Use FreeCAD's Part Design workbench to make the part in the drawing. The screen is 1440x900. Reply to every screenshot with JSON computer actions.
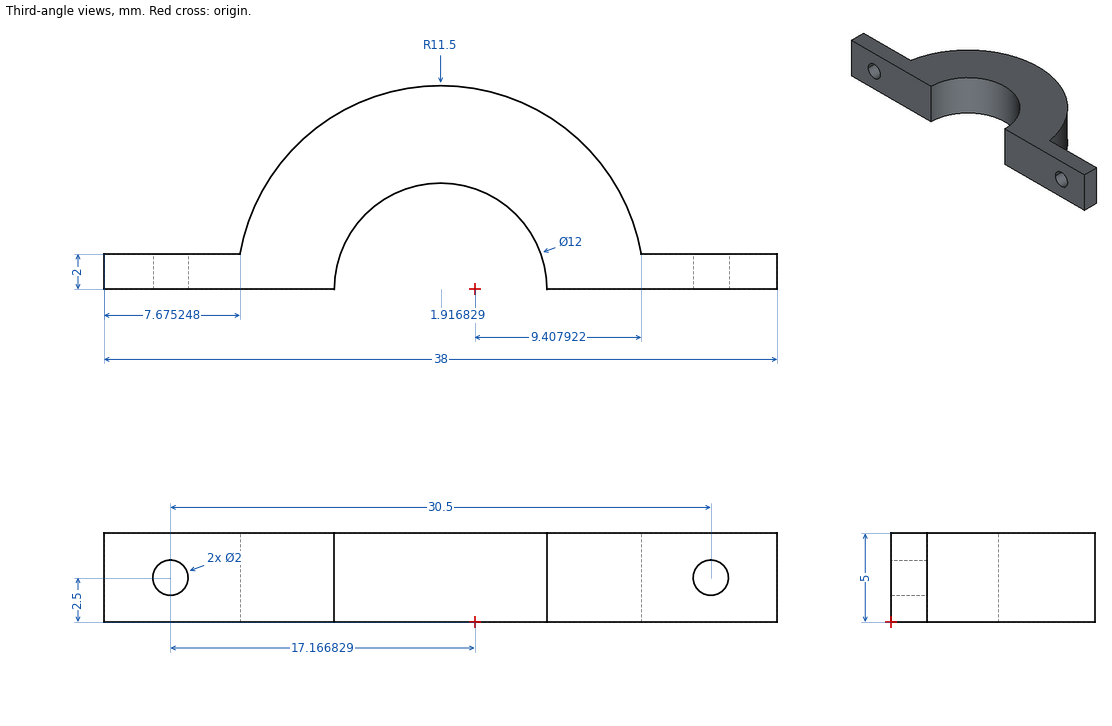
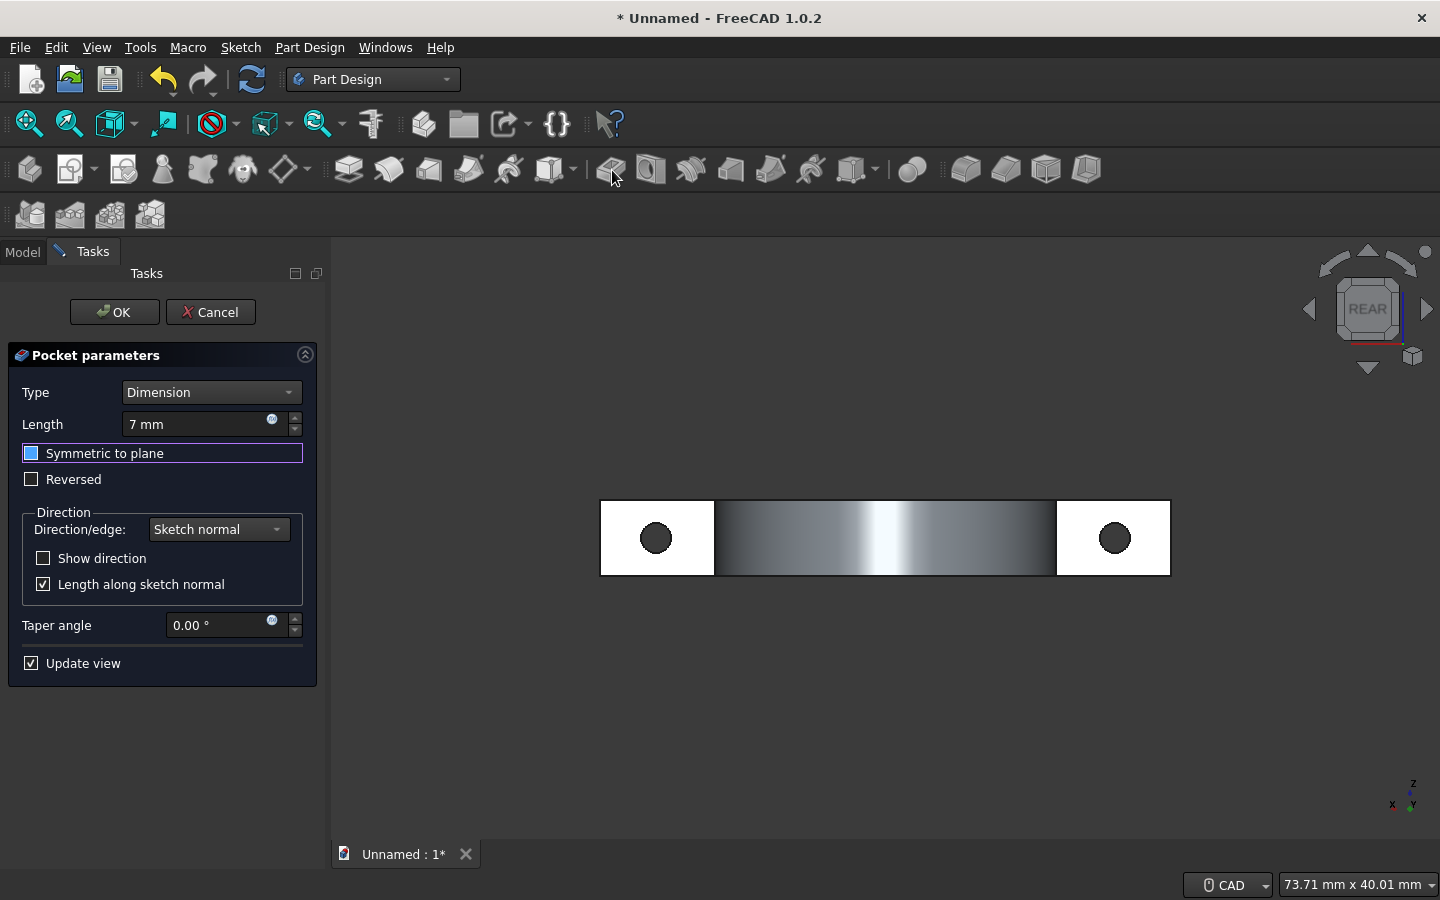
{"action": "left_click", "coordinate": [115, 312]}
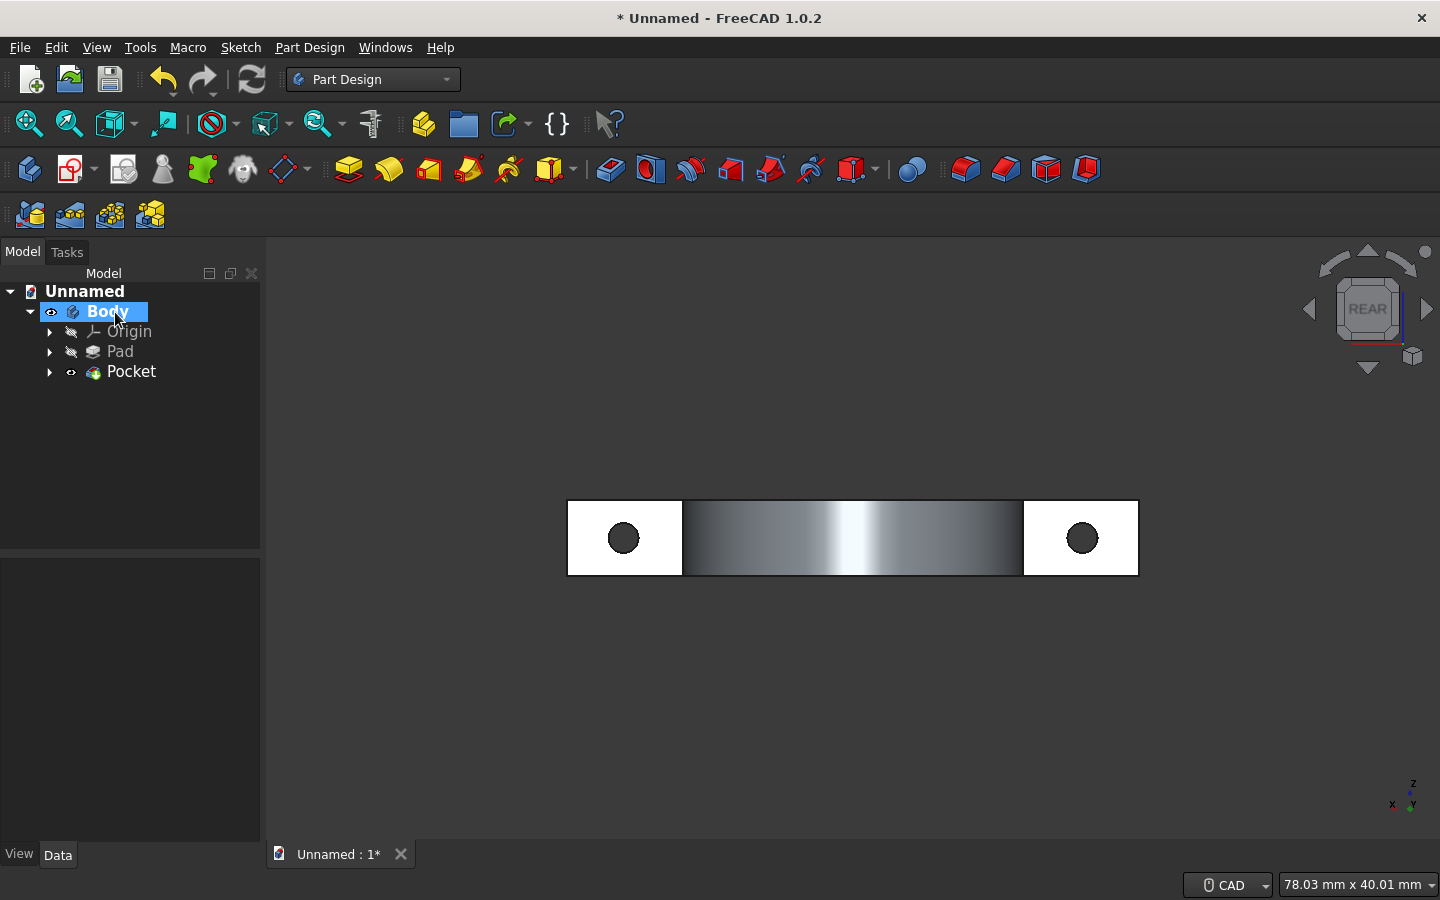
{"action": "key", "text": "0"}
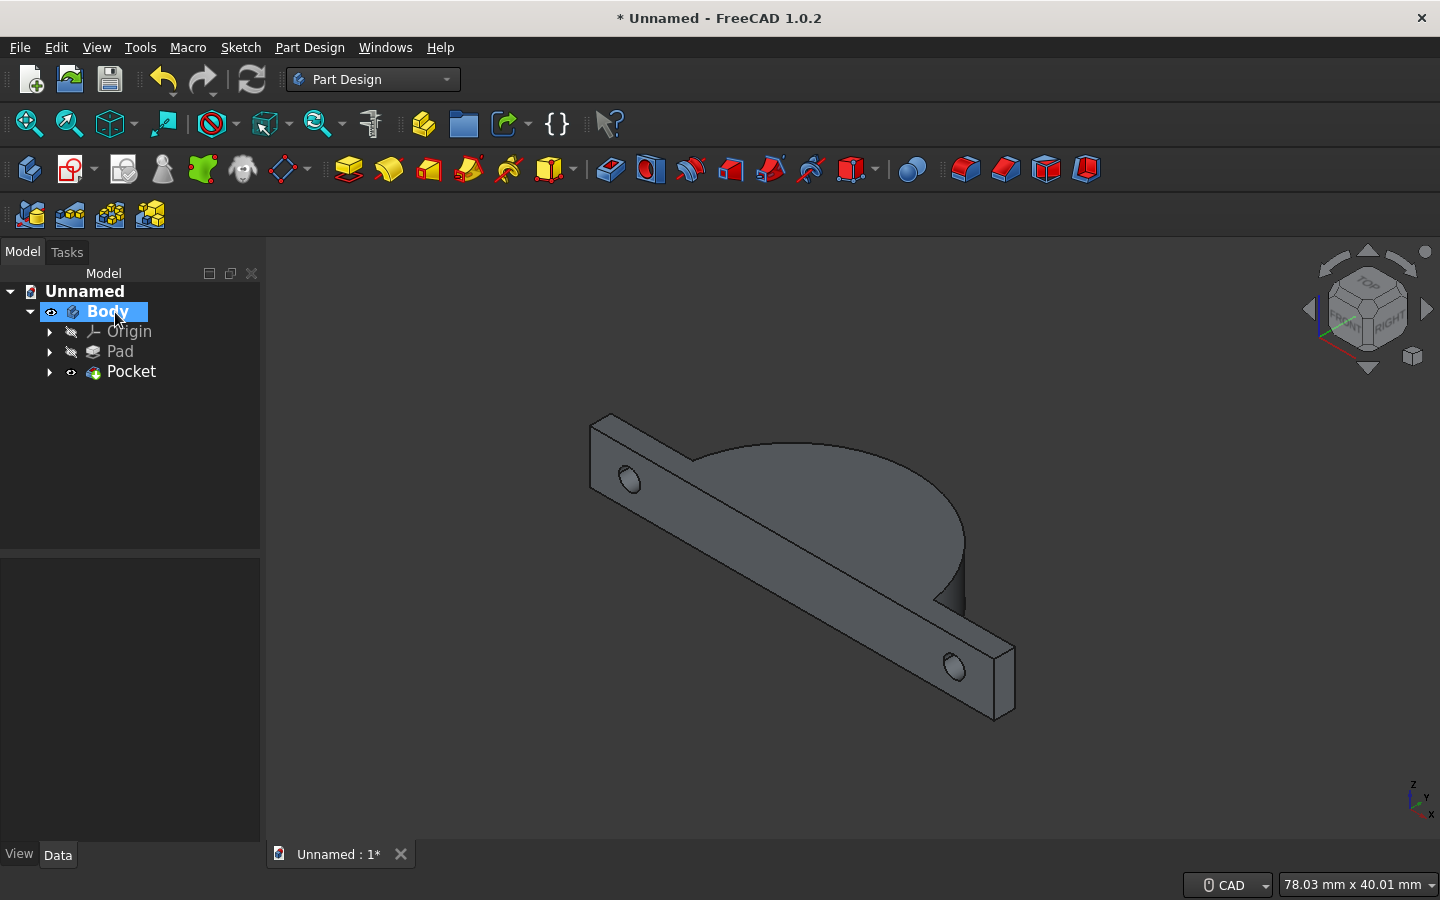
{"action": "left_click", "coordinate": [853, 506]}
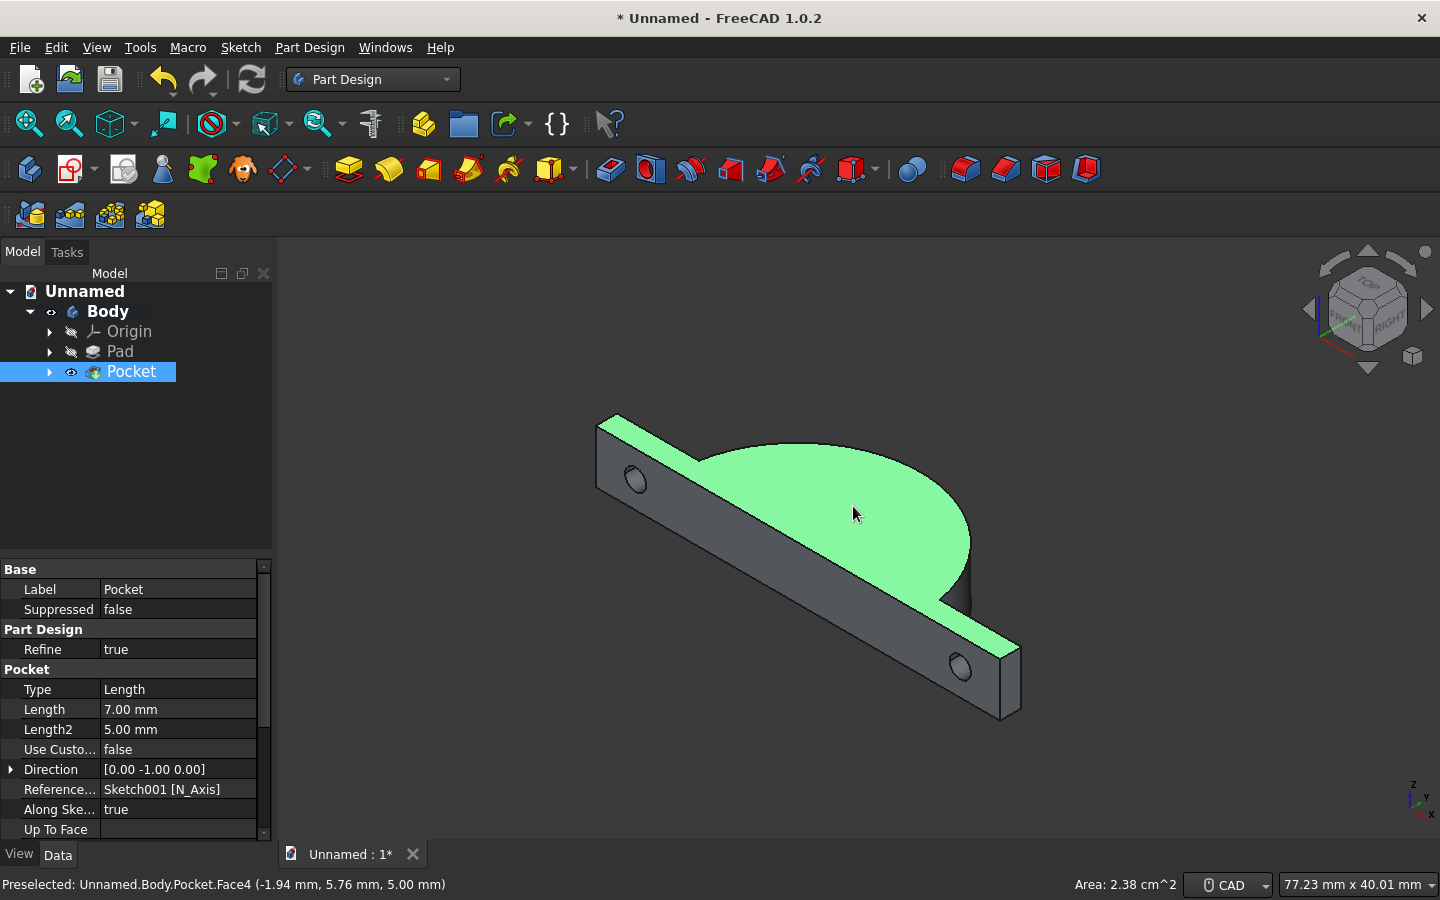
{"action": "left_click", "coordinate": [70, 170]}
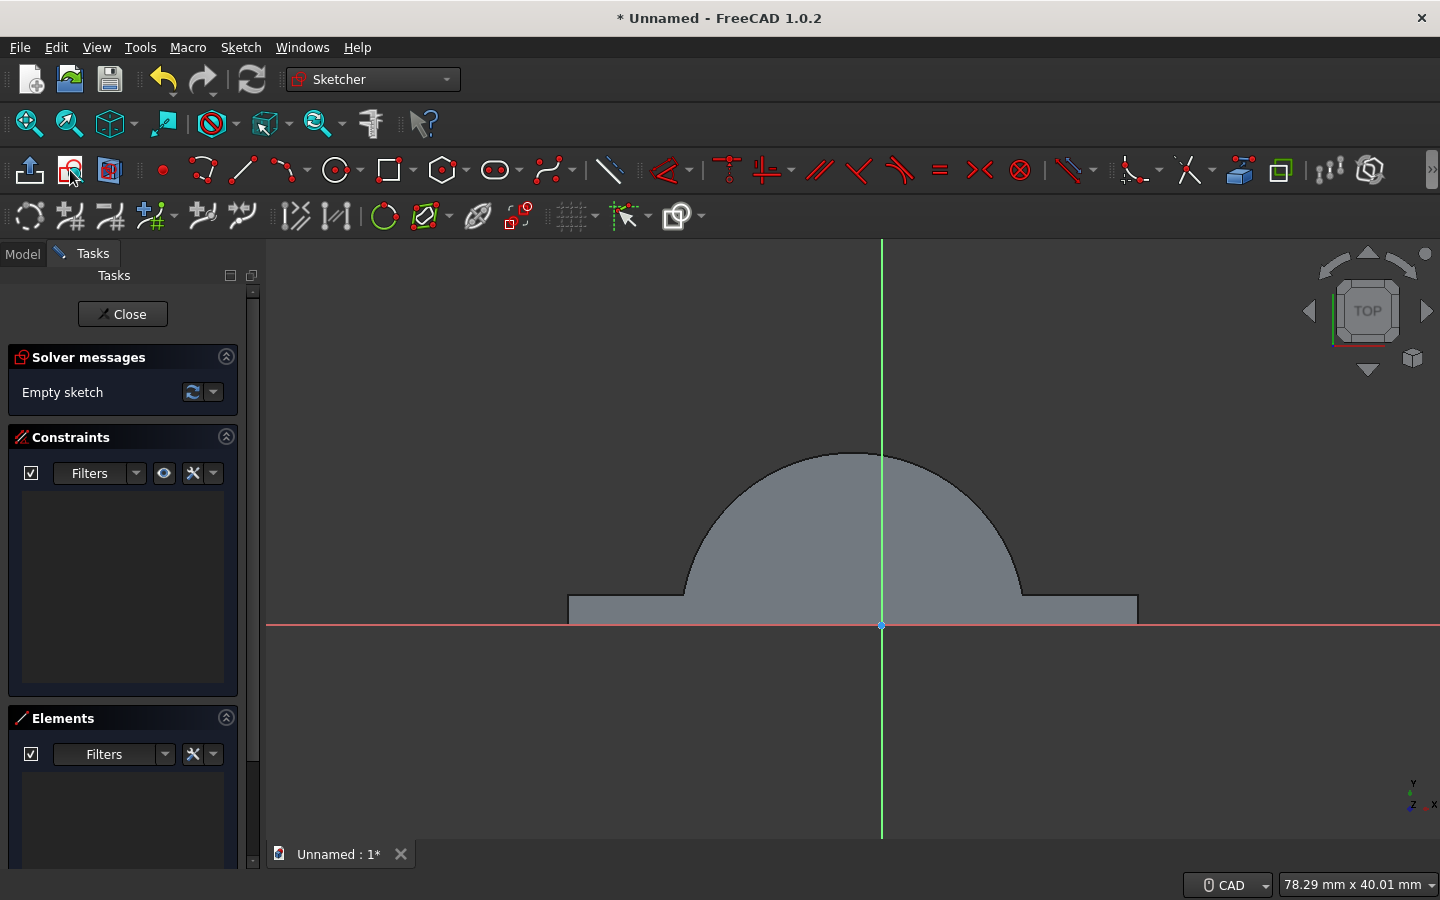
{"action": "scroll", "coordinate": [909, 695], "scroll_direction": "up", "scroll_amount": 4}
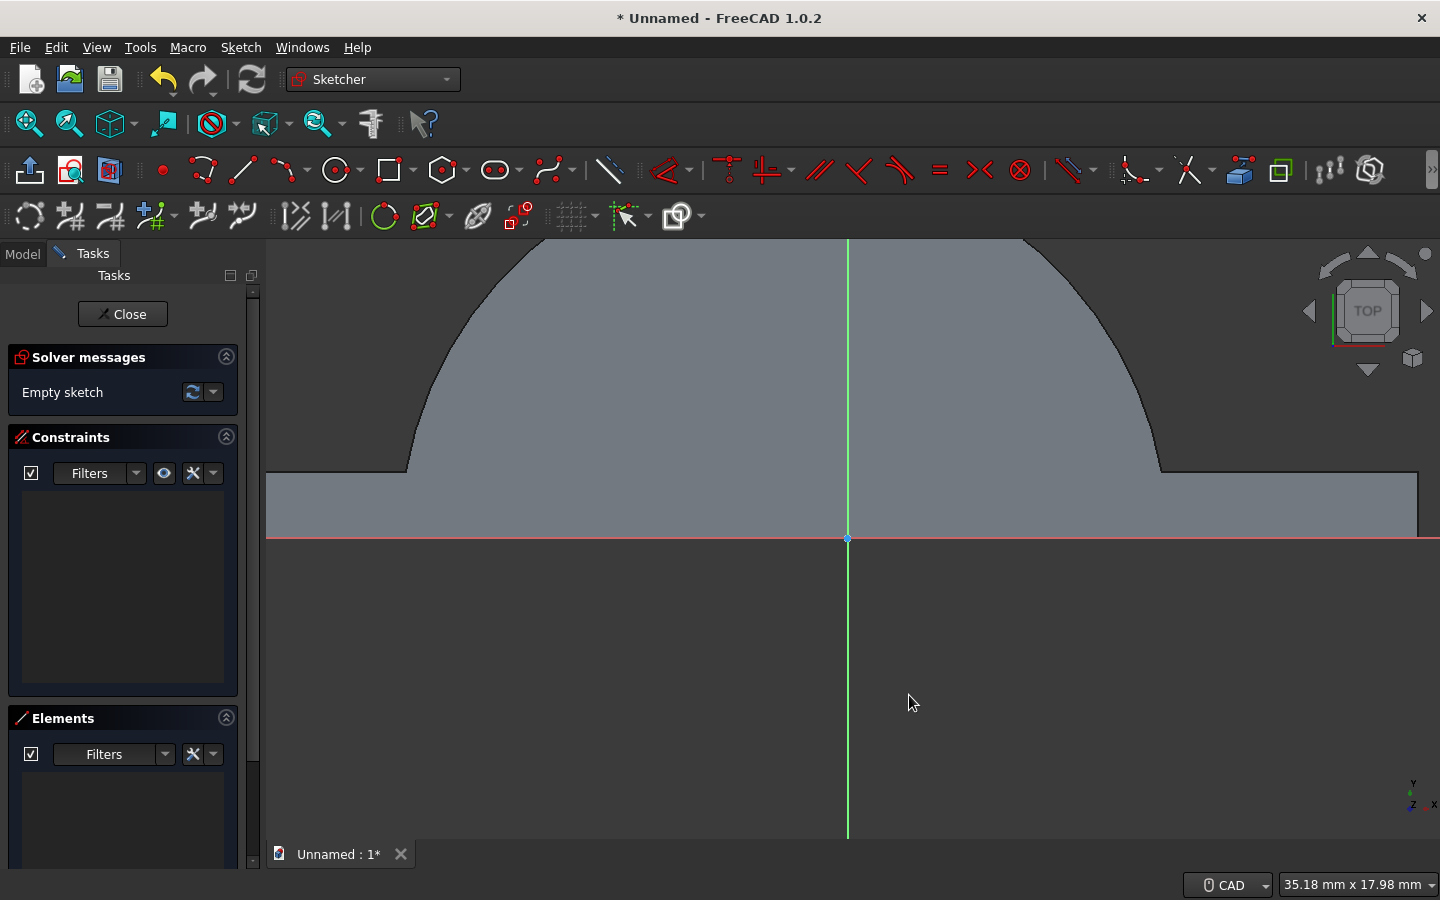
{"action": "key", "text": "g c"}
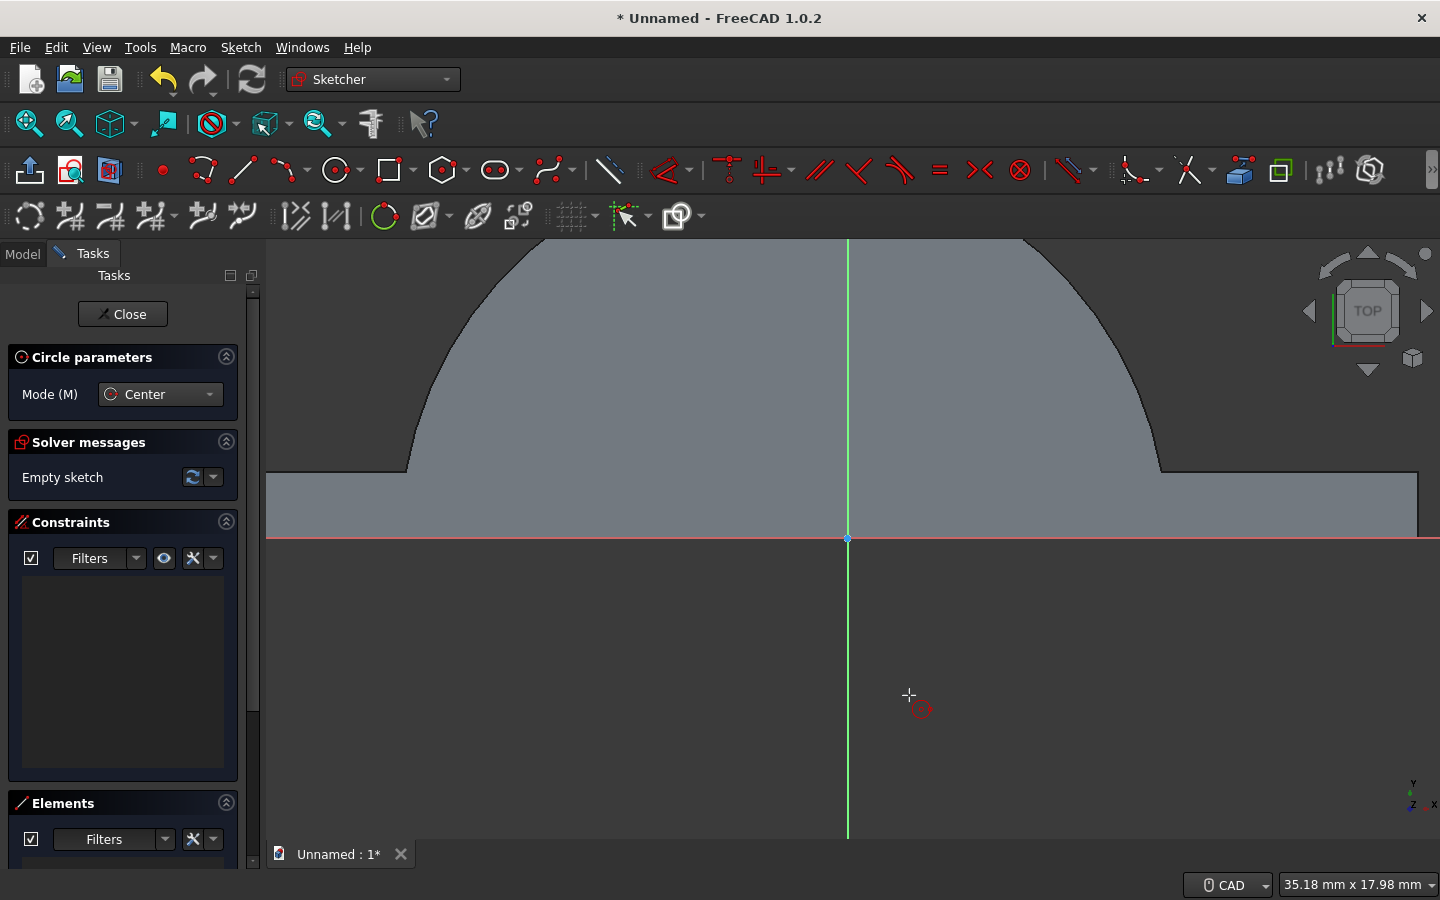
{"action": "left_click", "coordinate": [784, 538]}
{"action": "left_click", "coordinate": [925, 397]}
{"action": "key", "text": "Escape"}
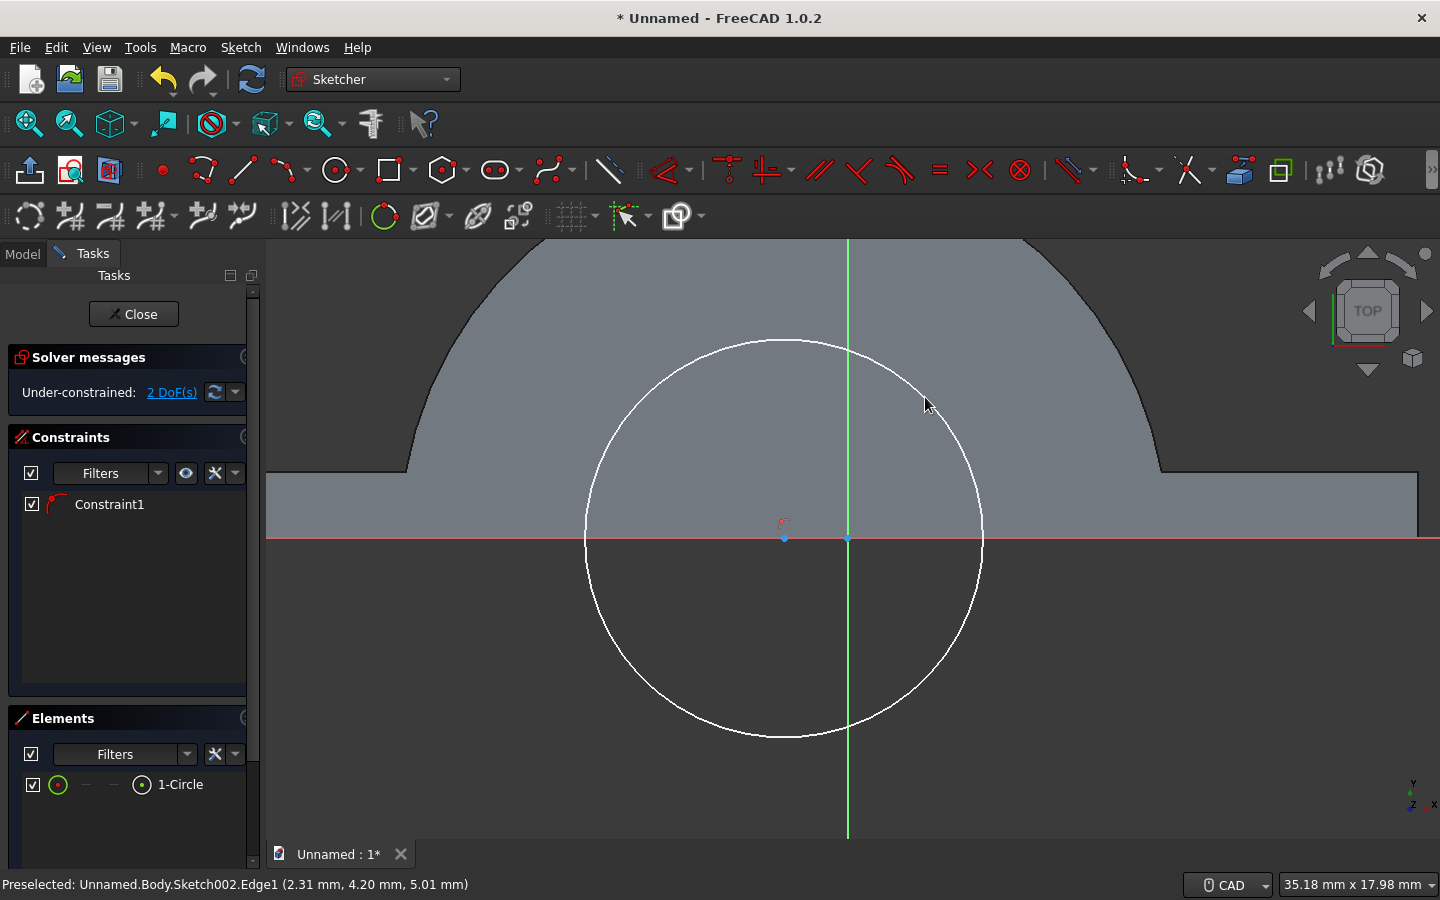
{"action": "left_click", "coordinate": [664, 170]}